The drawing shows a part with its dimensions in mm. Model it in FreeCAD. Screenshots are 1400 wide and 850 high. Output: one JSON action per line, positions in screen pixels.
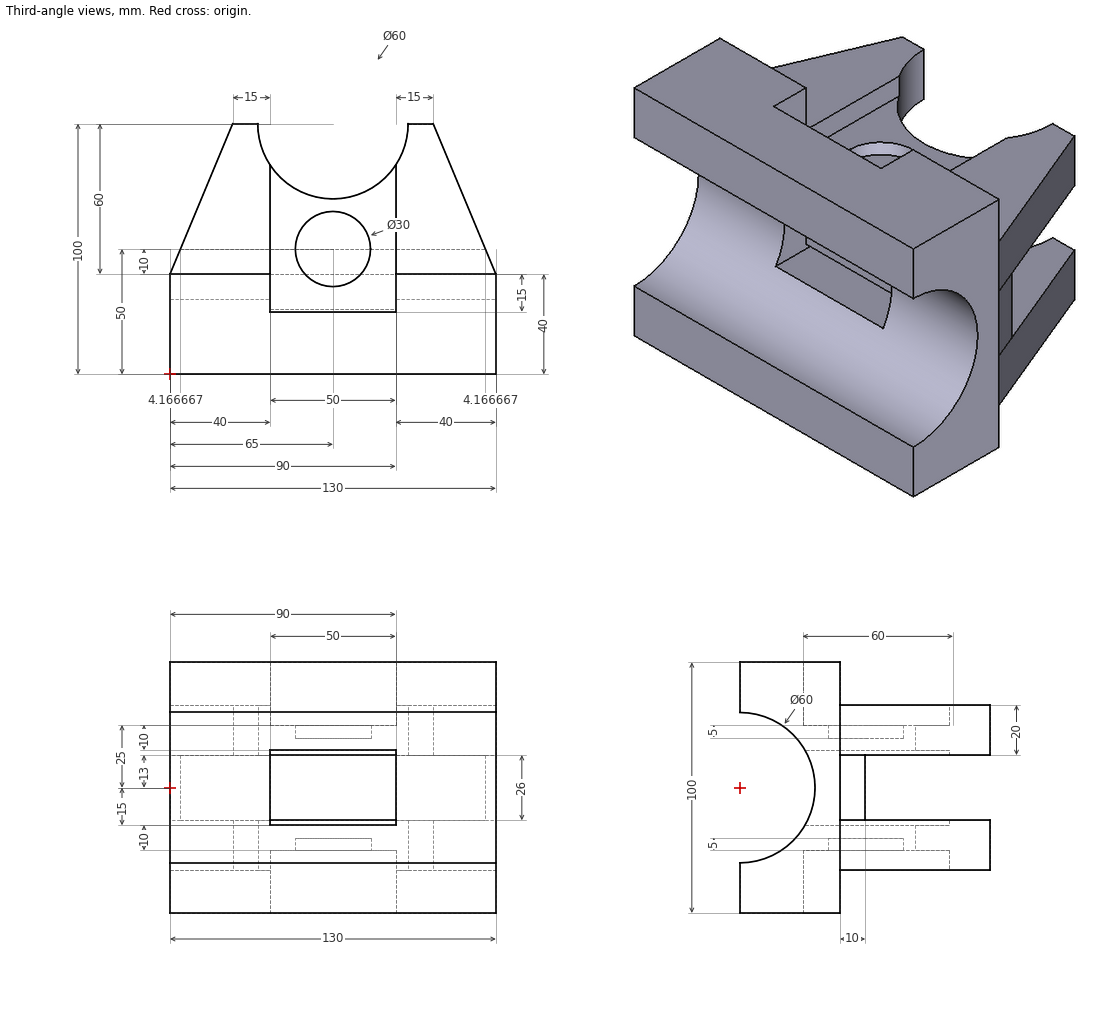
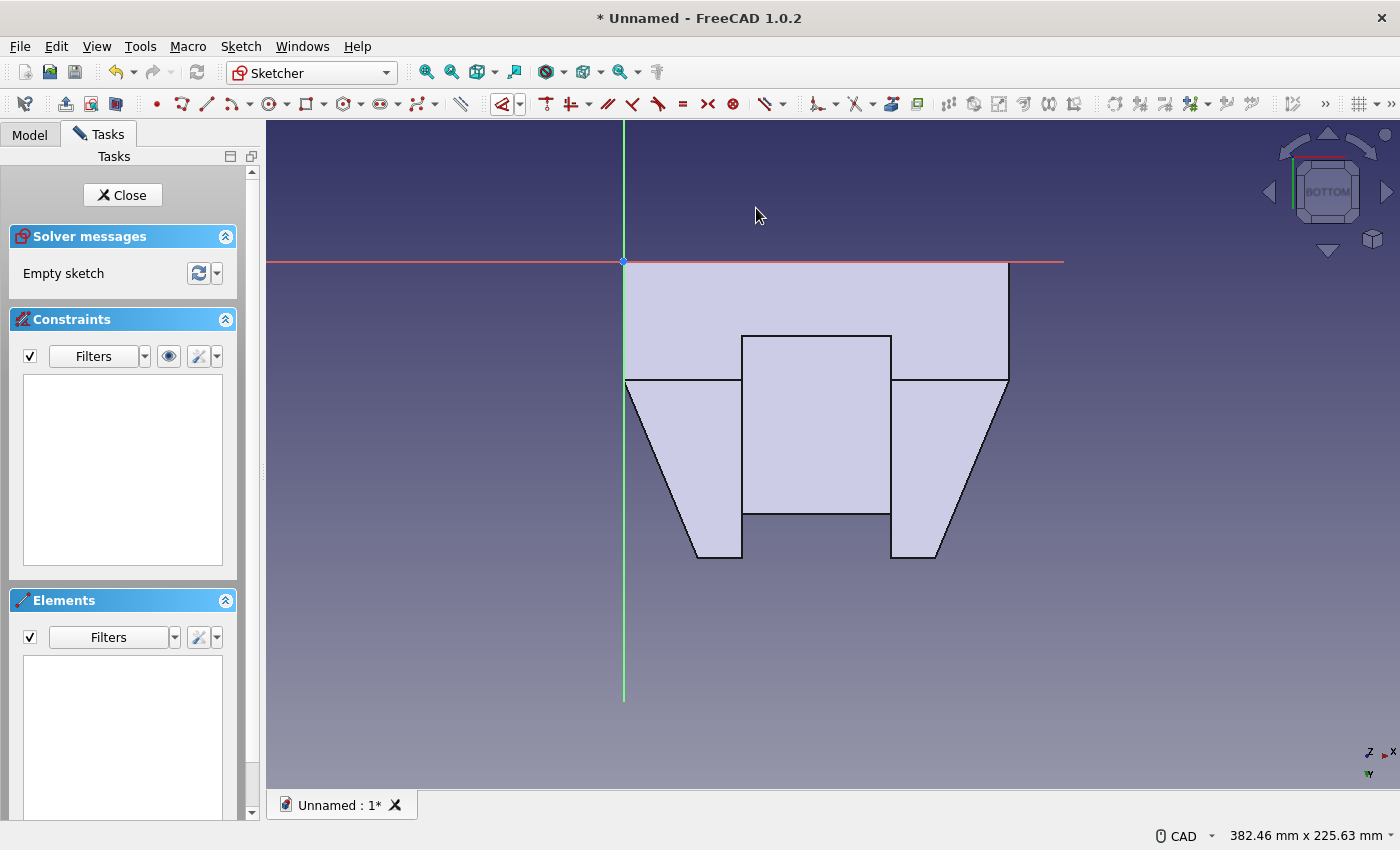
{"action": "left_click", "coordinate": [268, 104]}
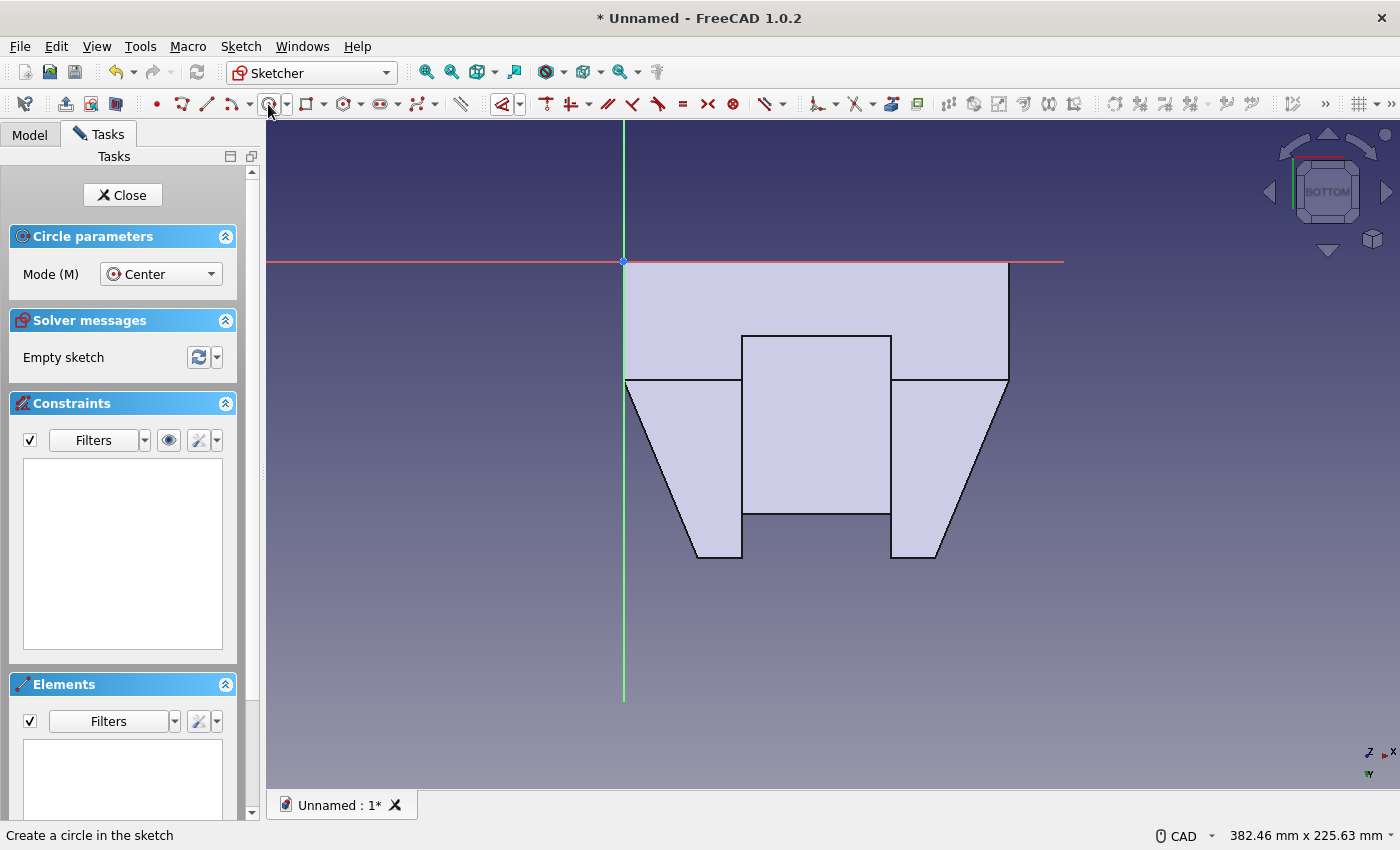
{"action": "left_click", "coordinate": [816, 558]}
{"action": "mouse_move", "coordinate": [879, 495]}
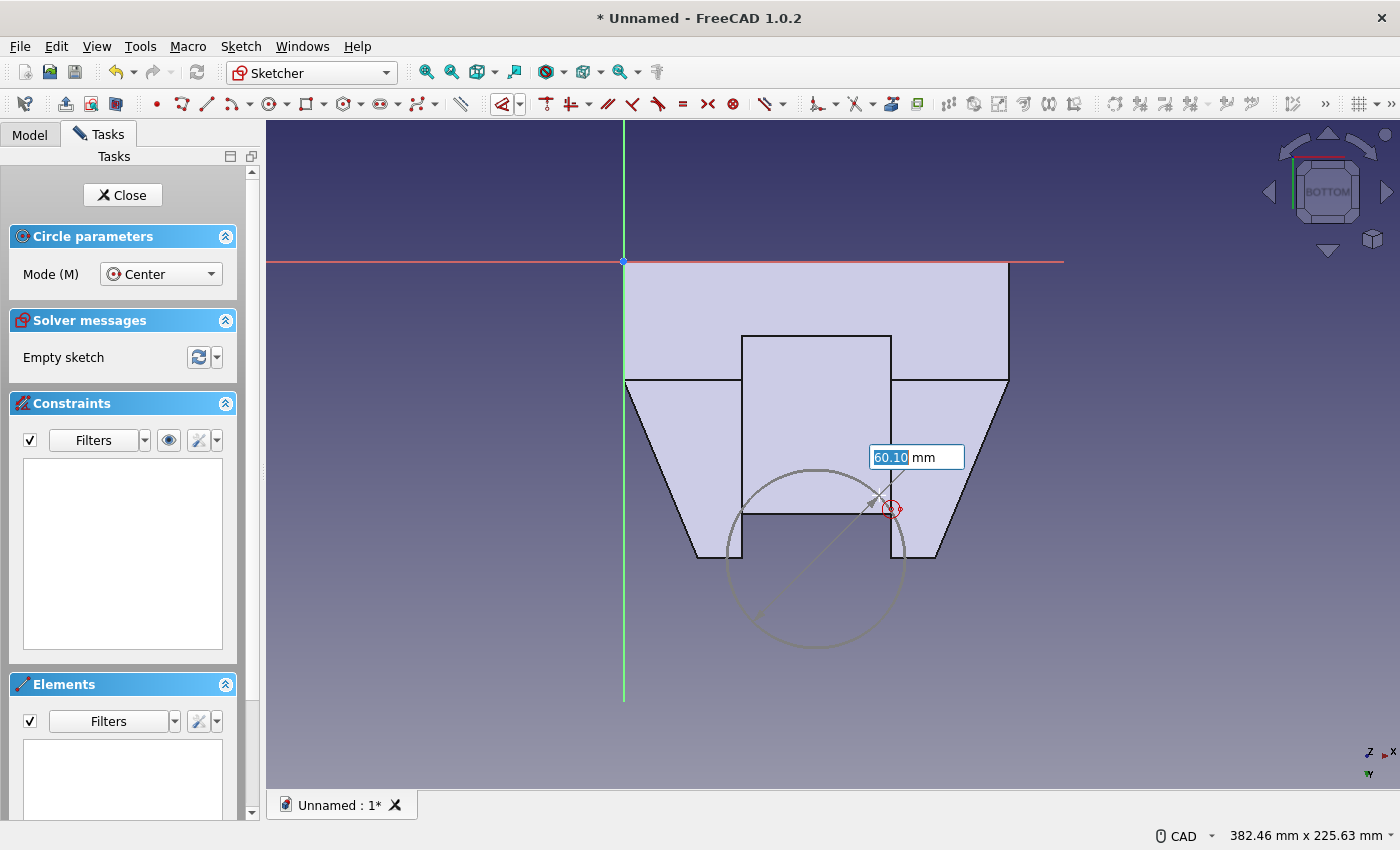
{"action": "type", "text": "60"}
{"action": "key", "text": "Return"}
{"action": "key", "text": "Escape"}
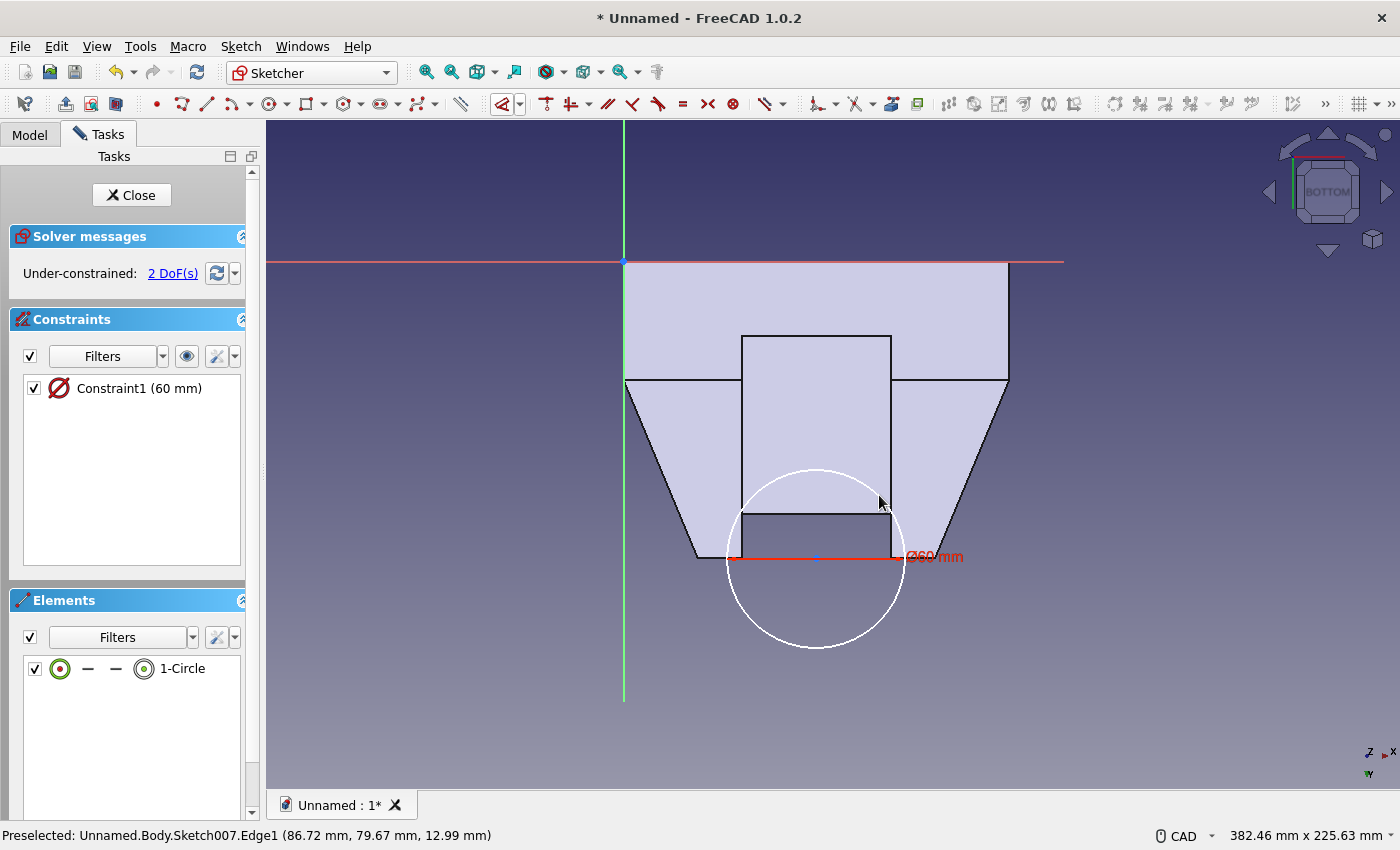
{"action": "left_click", "coordinate": [816, 559]}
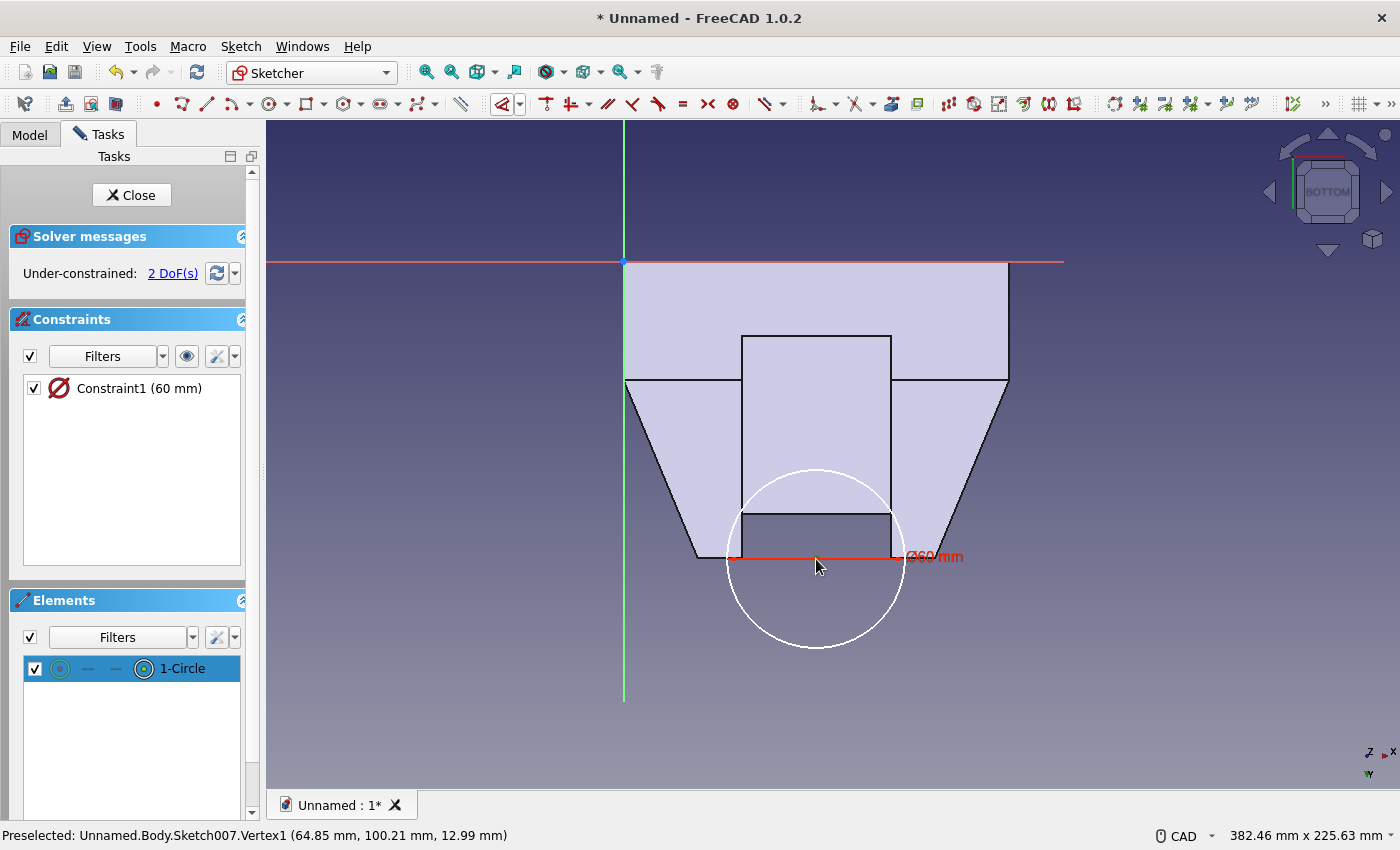
{"action": "left_click", "coordinate": [520, 104]}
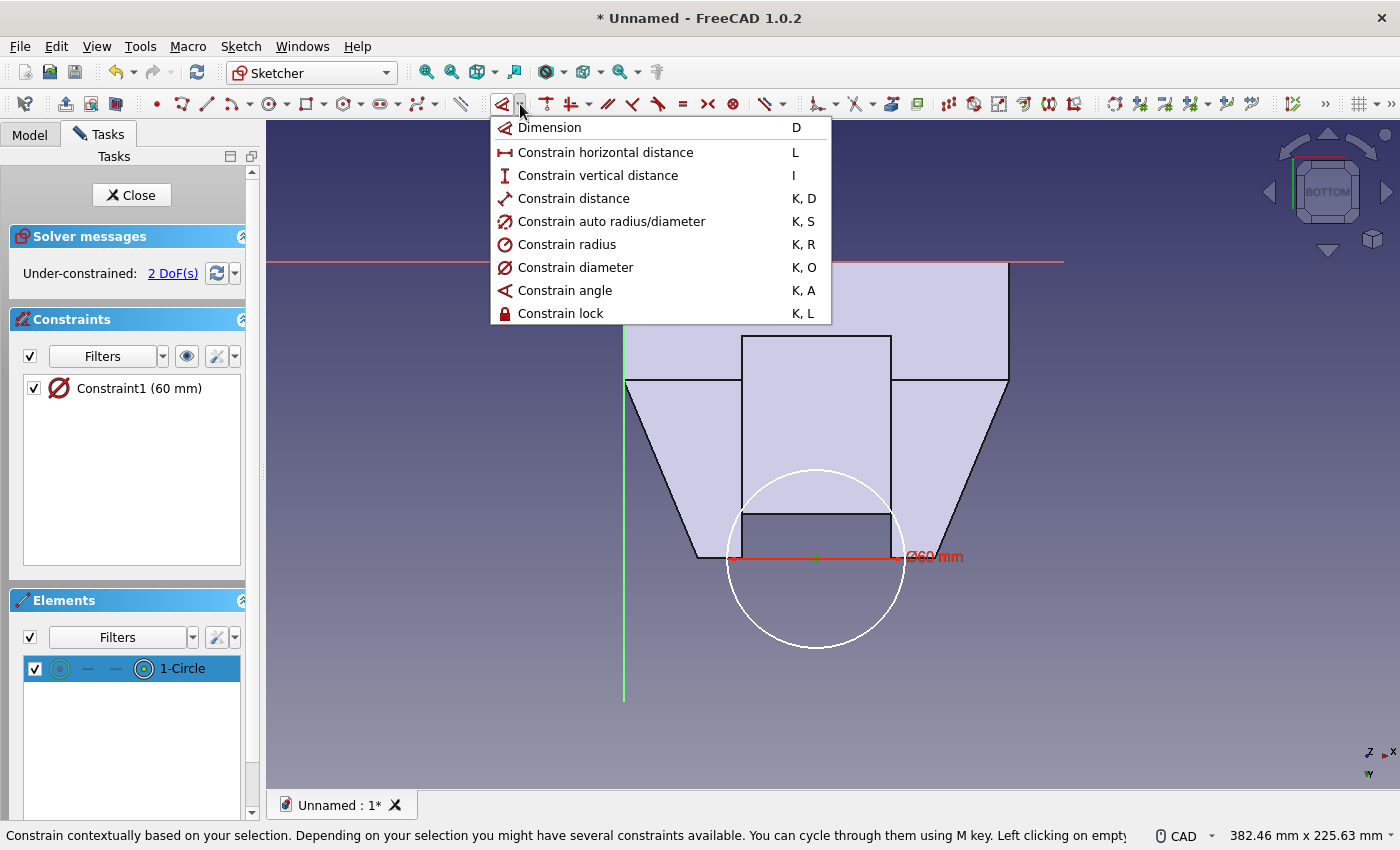
{"action": "left_click", "coordinate": [661, 152]}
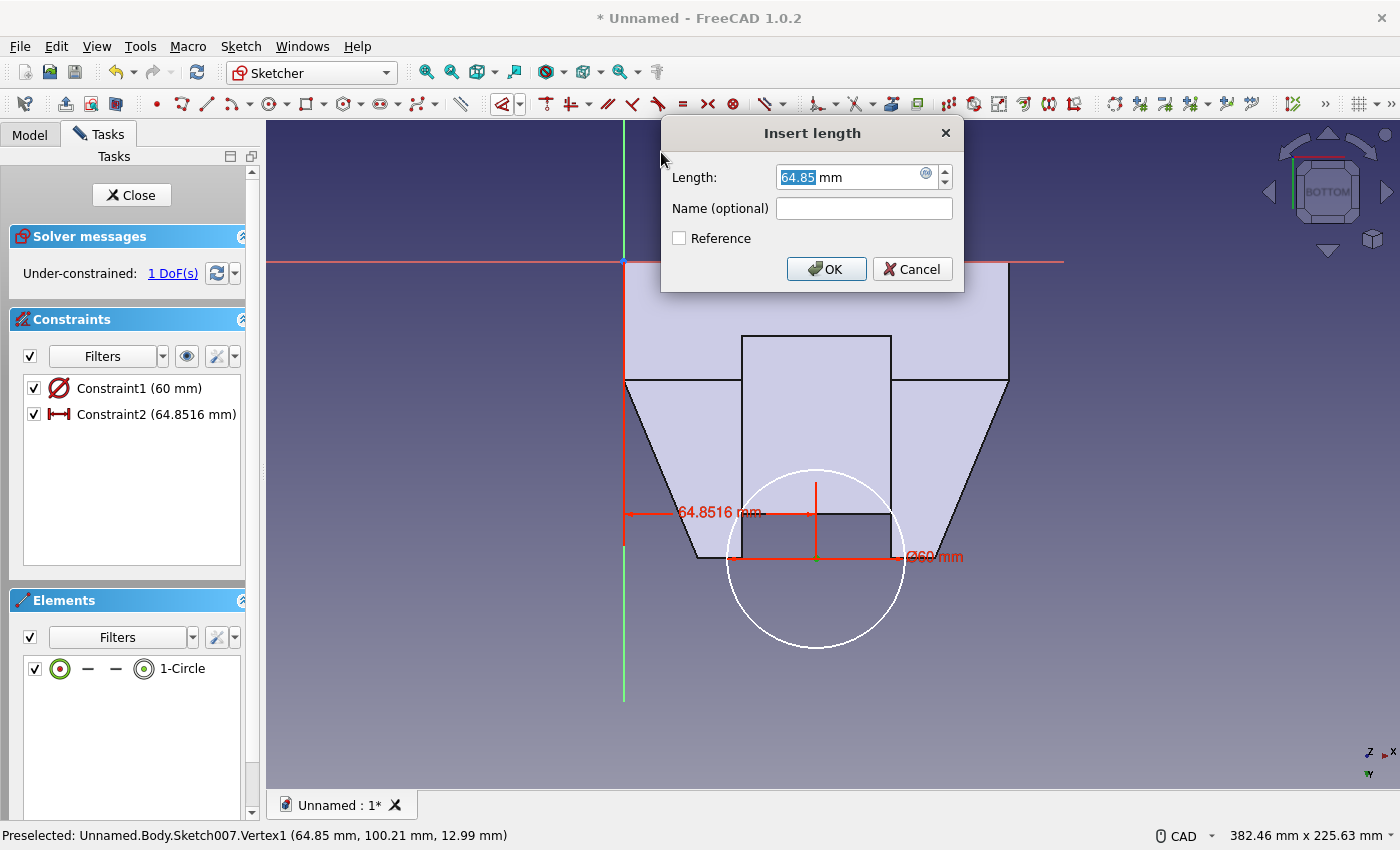
{"action": "type", "text": "65"}
{"action": "key", "text": "Return"}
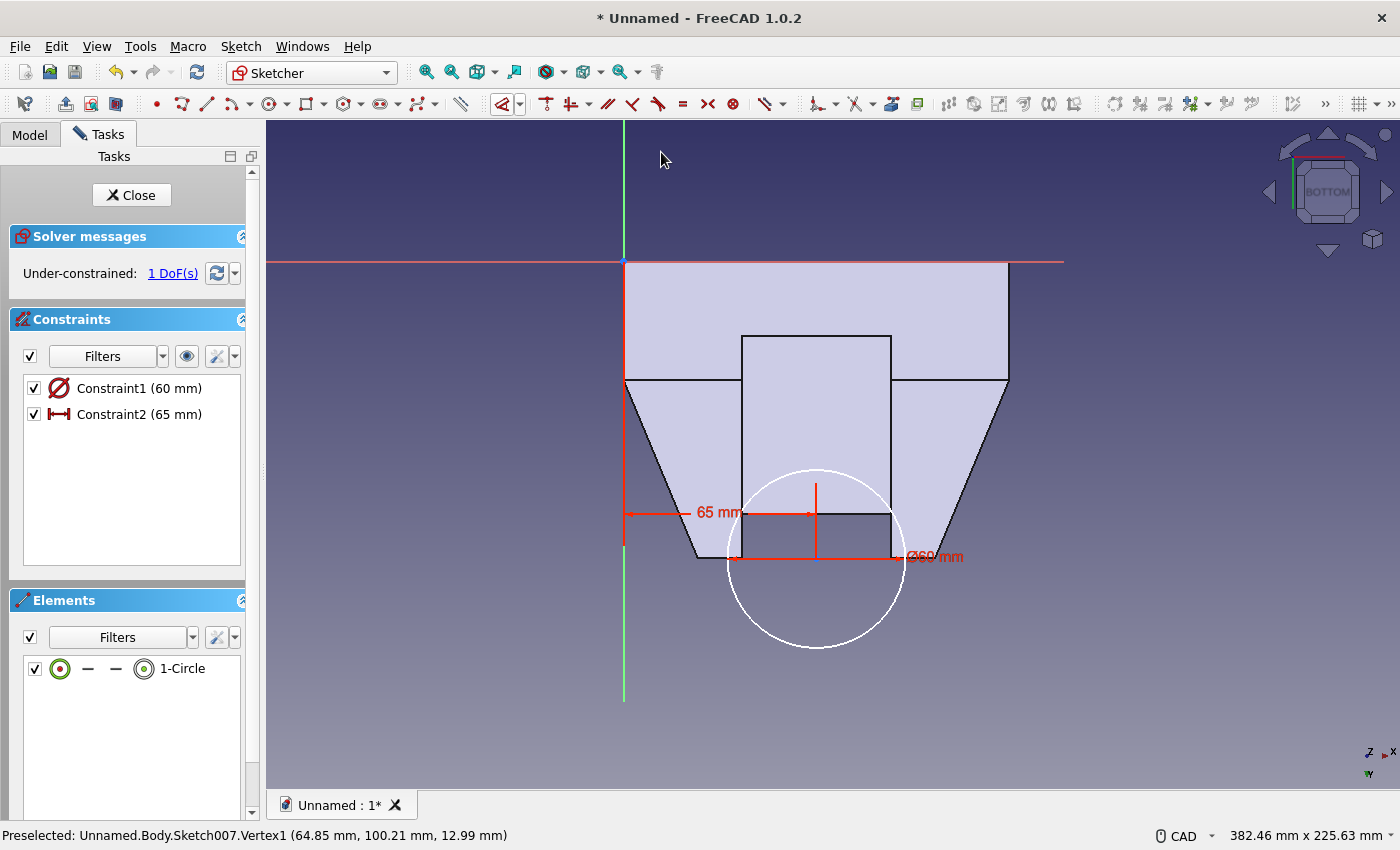
{"action": "left_click", "coordinate": [816, 559]}